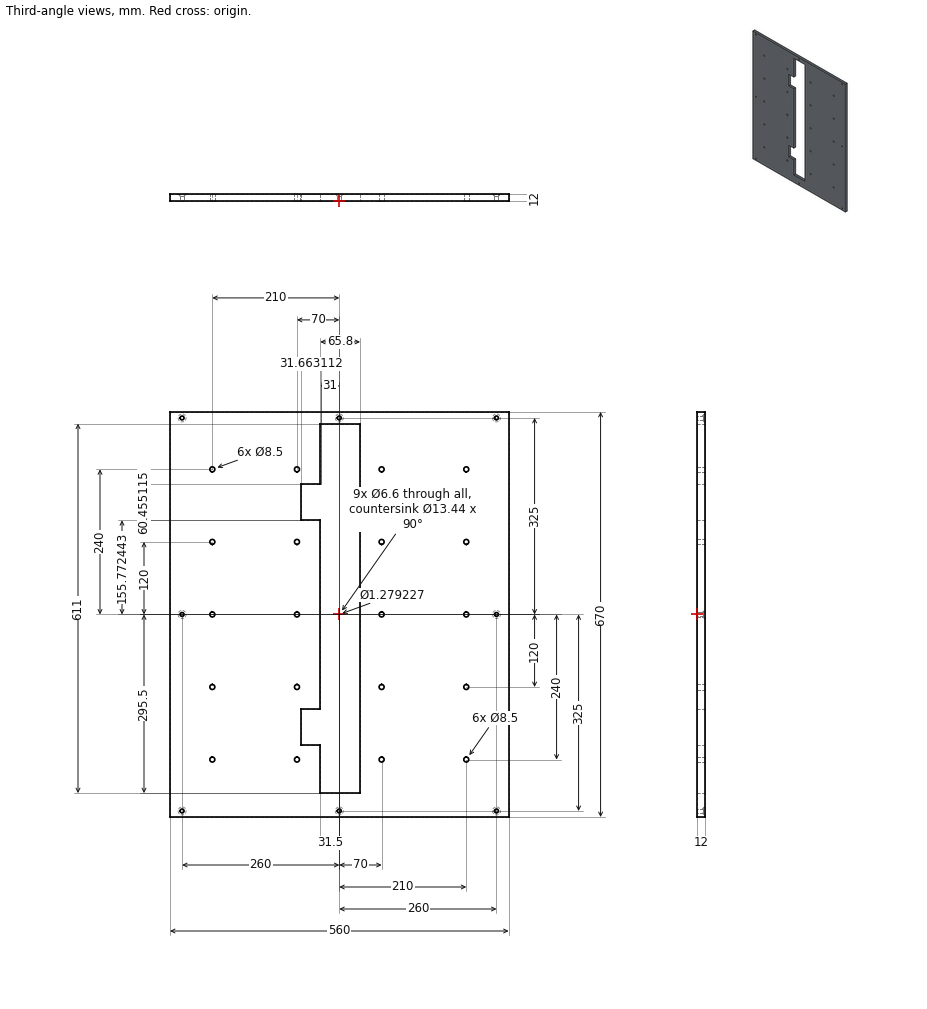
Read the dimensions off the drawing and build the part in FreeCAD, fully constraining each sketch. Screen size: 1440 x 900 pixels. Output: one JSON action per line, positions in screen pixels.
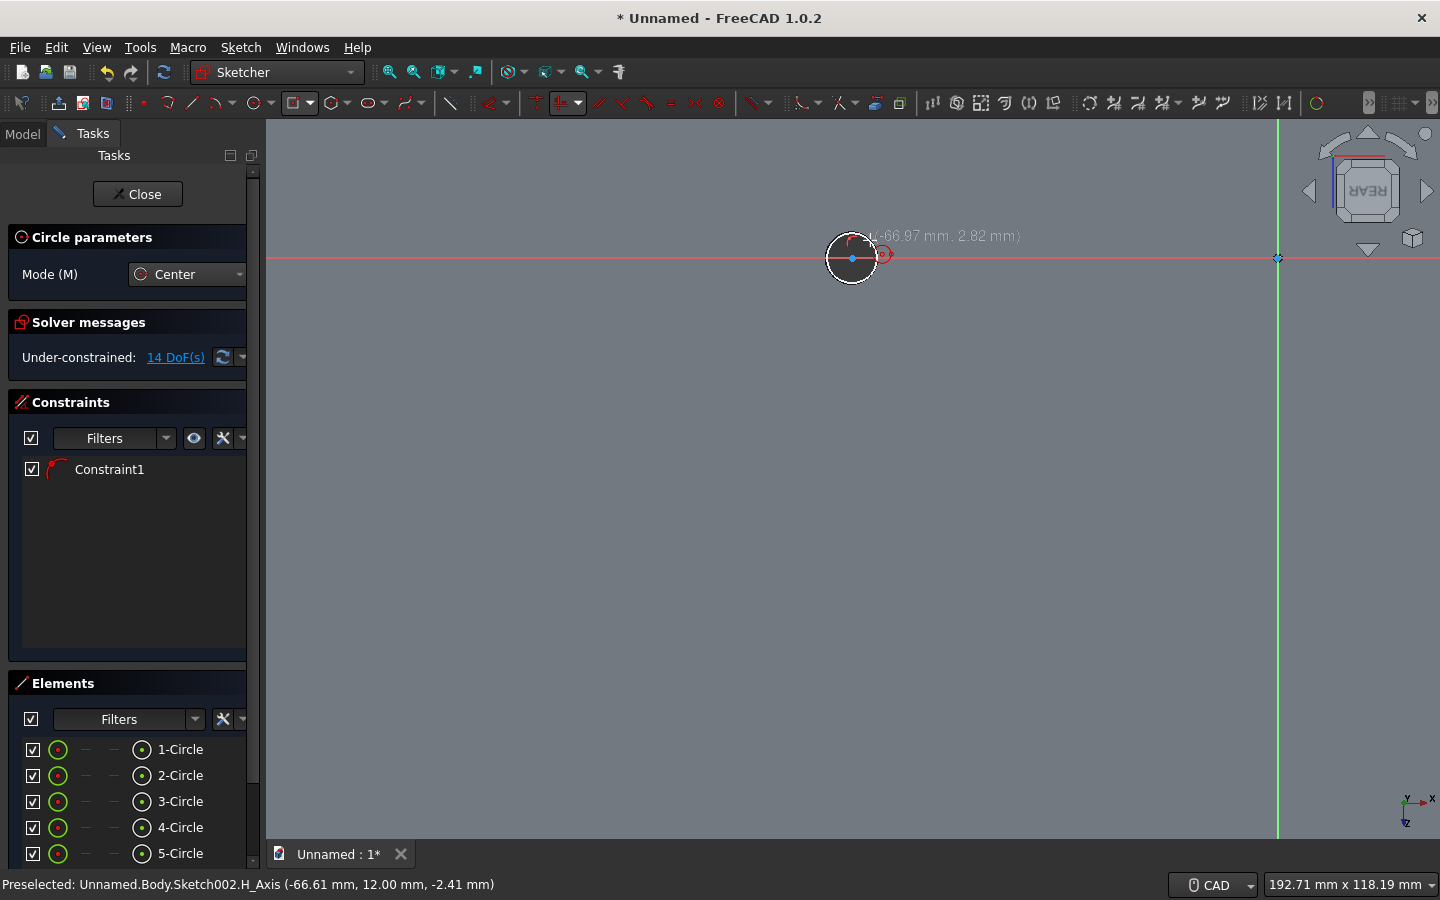
{"action": "scroll", "coordinate": [852, 259], "scroll_direction": "down", "scroll_amount": 6}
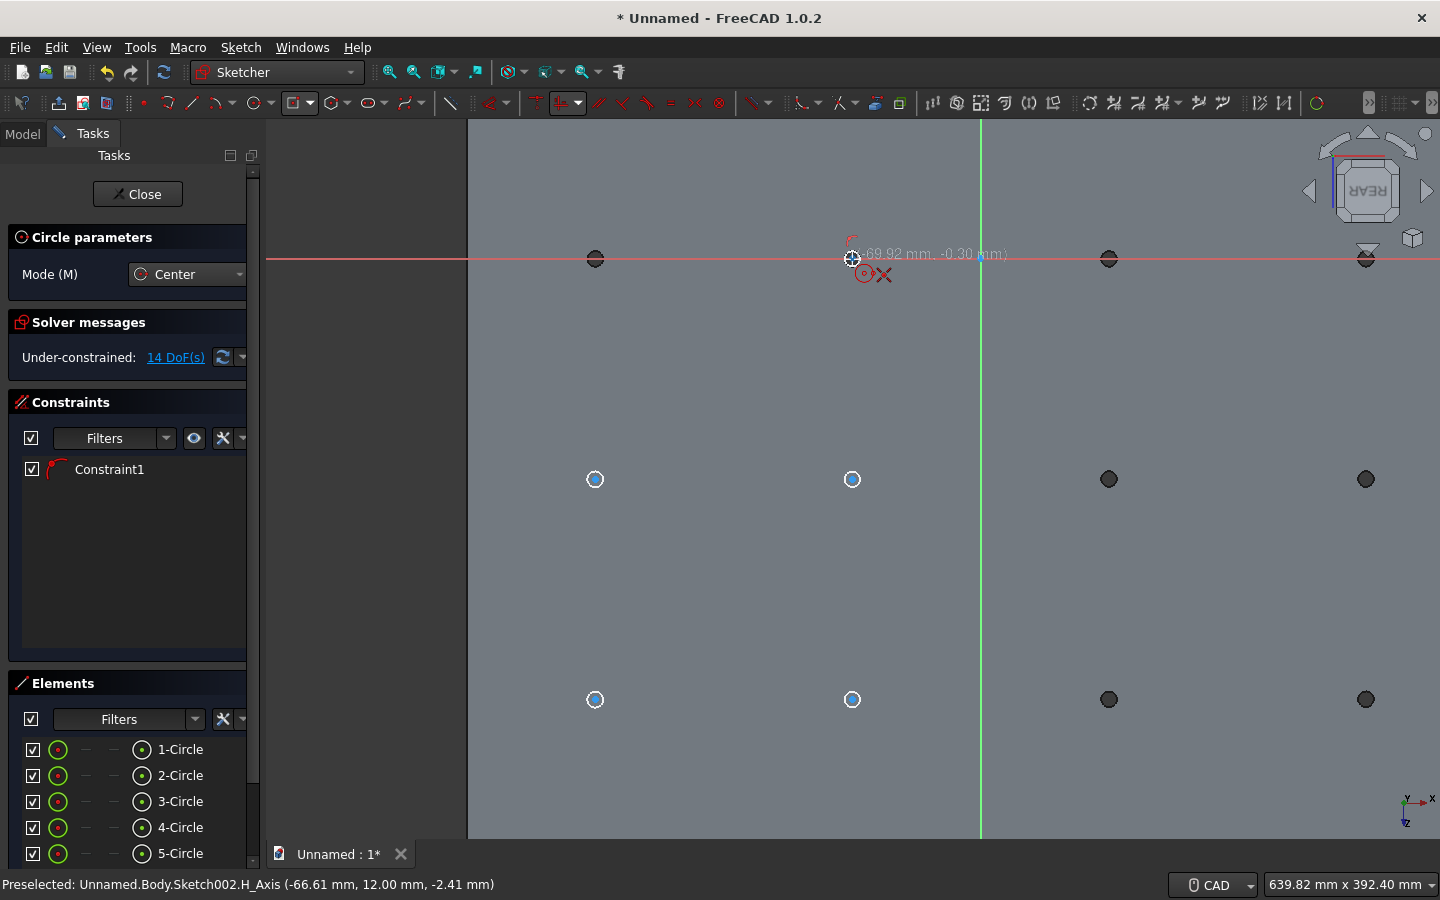
{"action": "scroll", "coordinate": [595, 259], "scroll_direction": "up", "scroll_amount": 6}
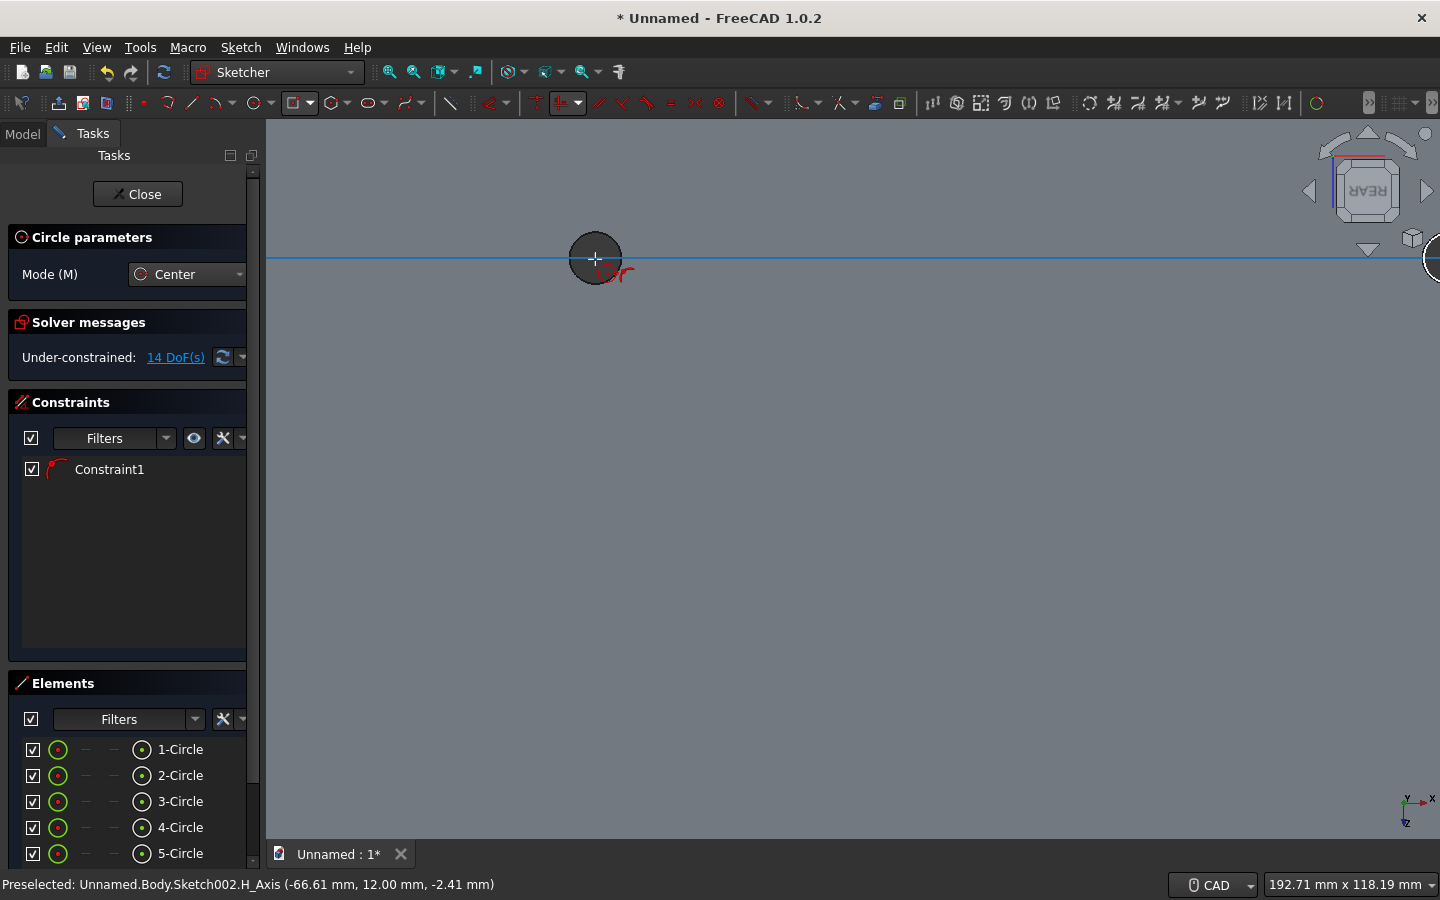
{"action": "left_click", "coordinate": [595, 258]}
{"action": "left_click", "coordinate": [614, 240]}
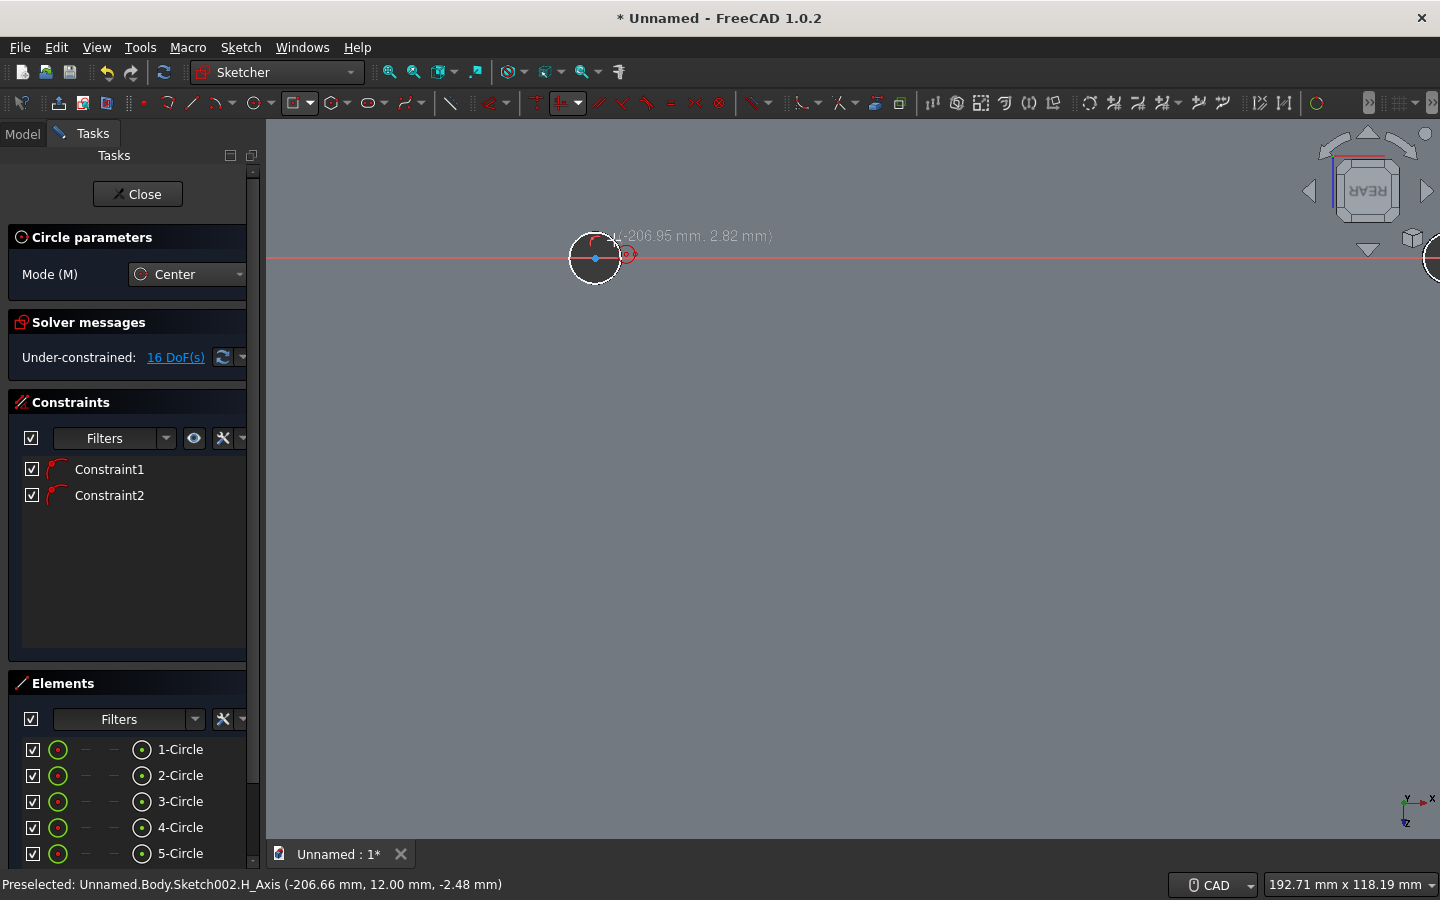
{"action": "scroll", "coordinate": [595, 259], "scroll_direction": "down", "scroll_amount": 6}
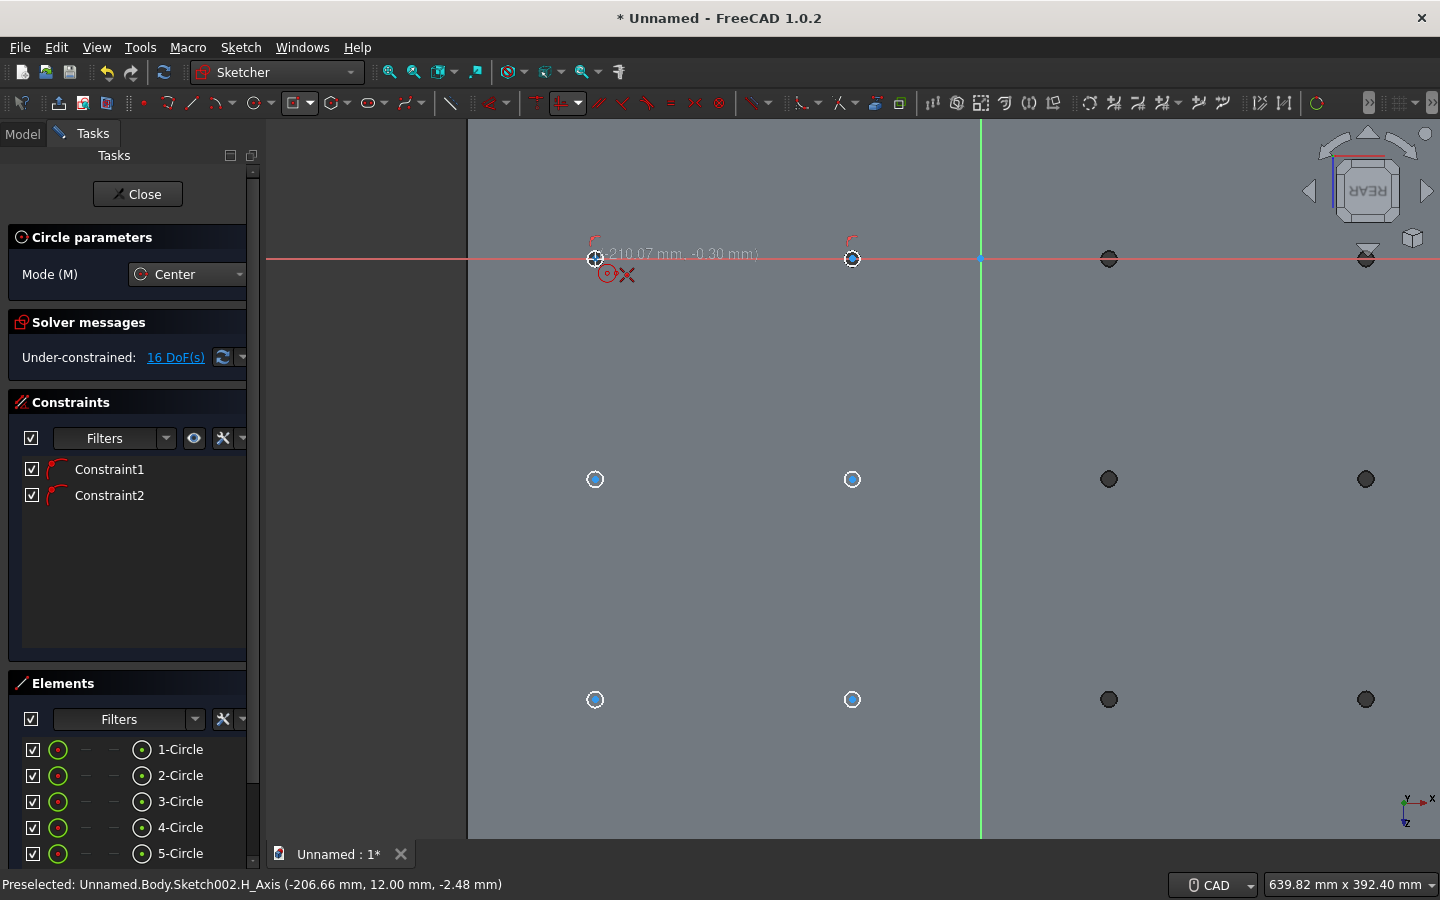
{"action": "scroll", "coordinate": [981, 259], "scroll_direction": "up", "scroll_amount": 15}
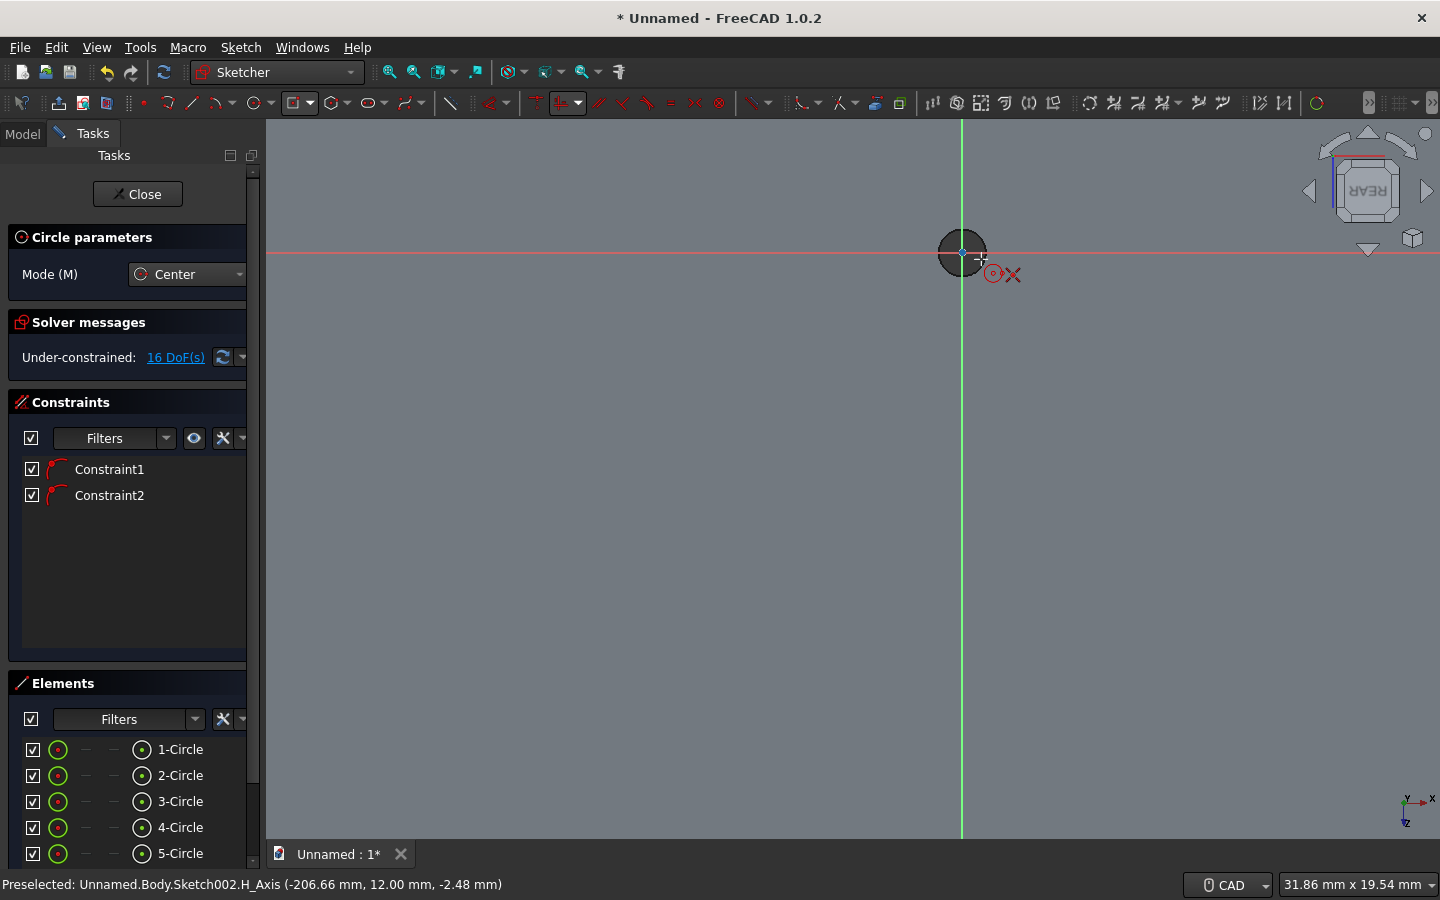
{"action": "scroll", "coordinate": [981, 259], "scroll_direction": "down", "scroll_amount": 15}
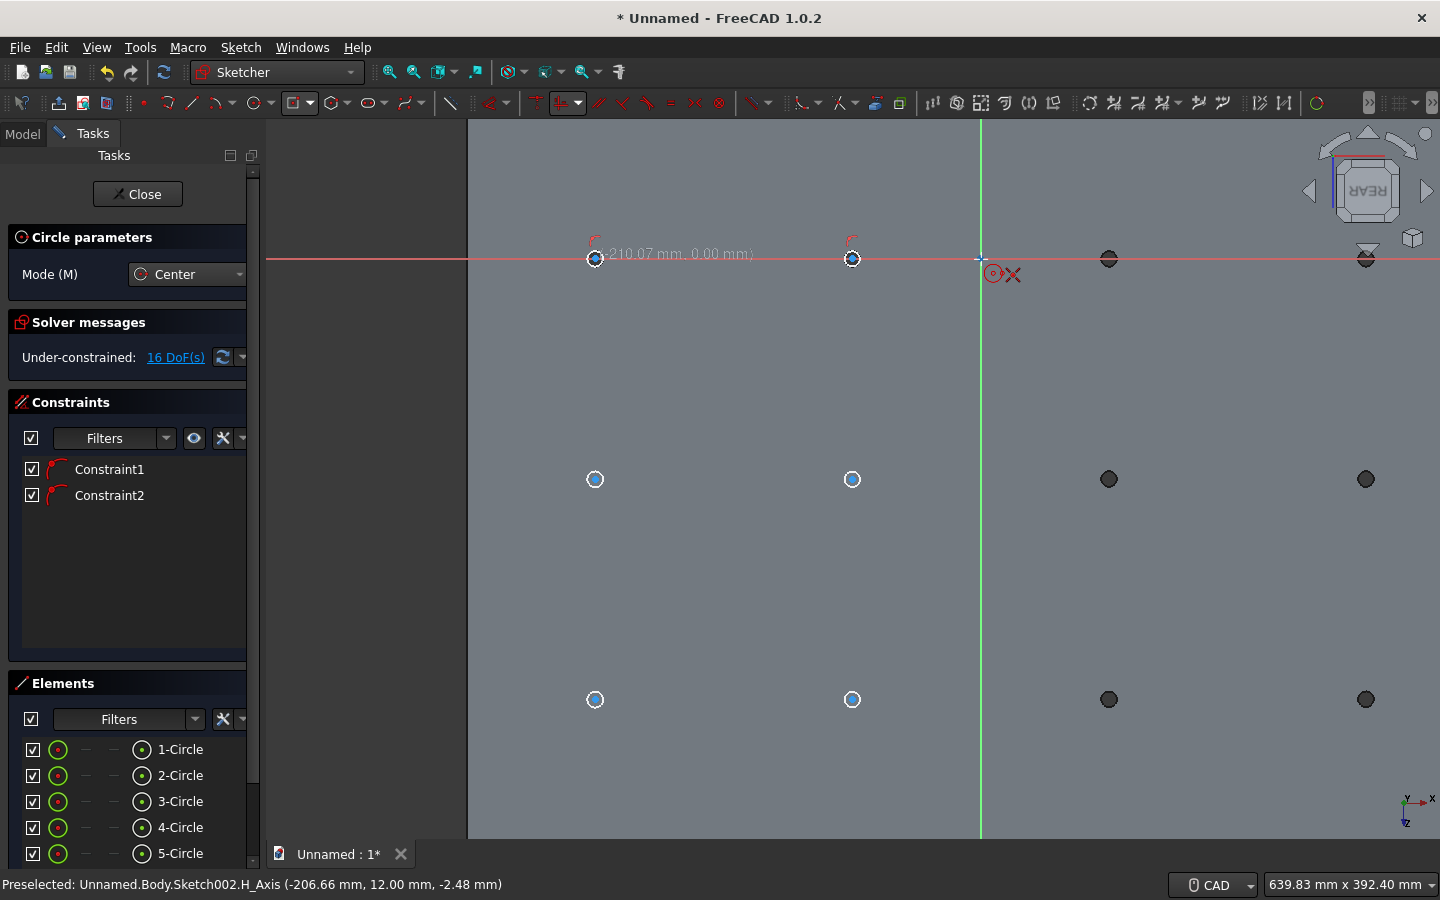
{"action": "left_click", "coordinate": [981, 259]}